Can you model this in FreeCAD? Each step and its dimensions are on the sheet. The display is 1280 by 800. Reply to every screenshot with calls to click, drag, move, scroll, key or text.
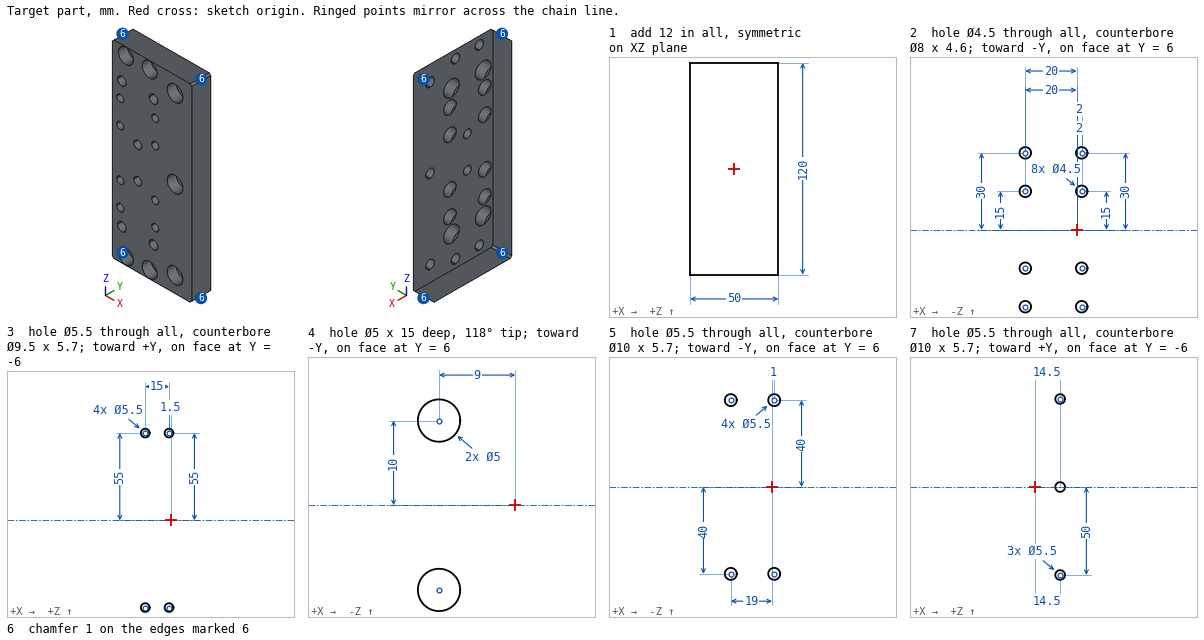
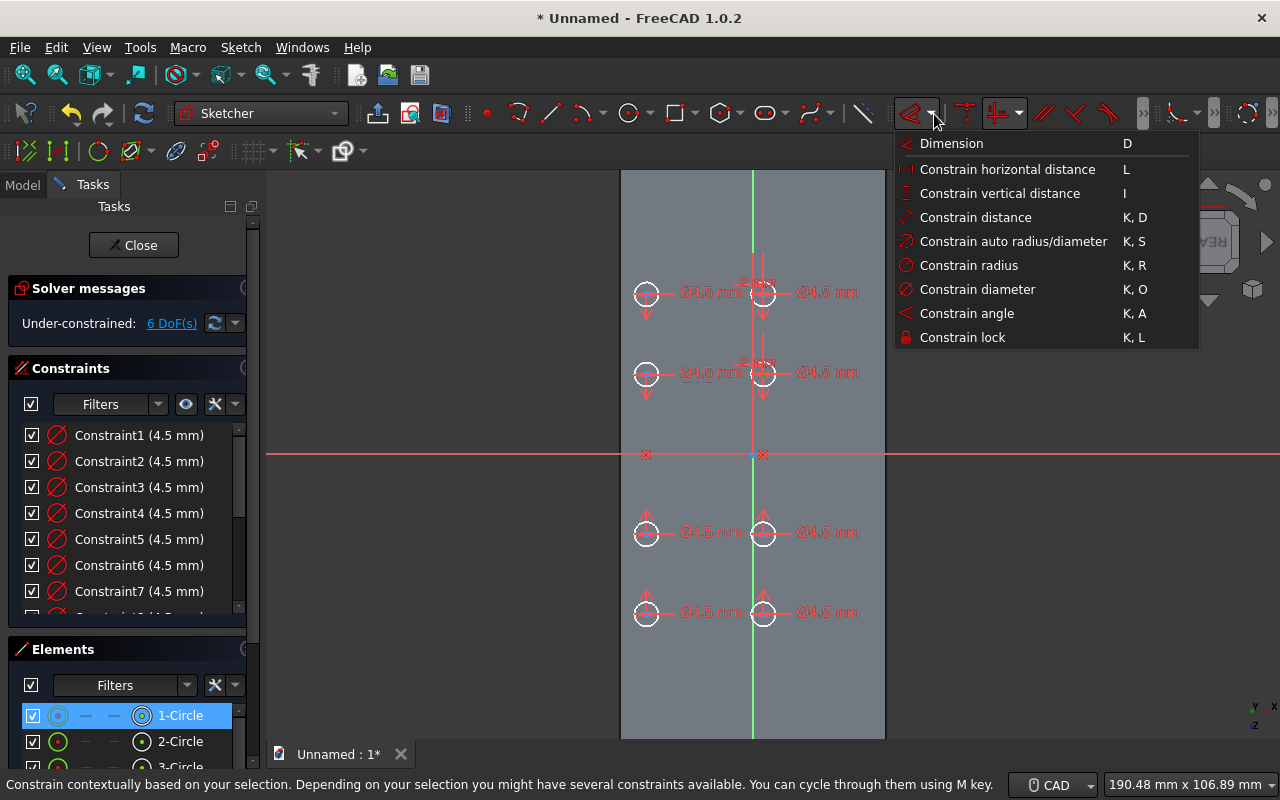
click(1047, 193)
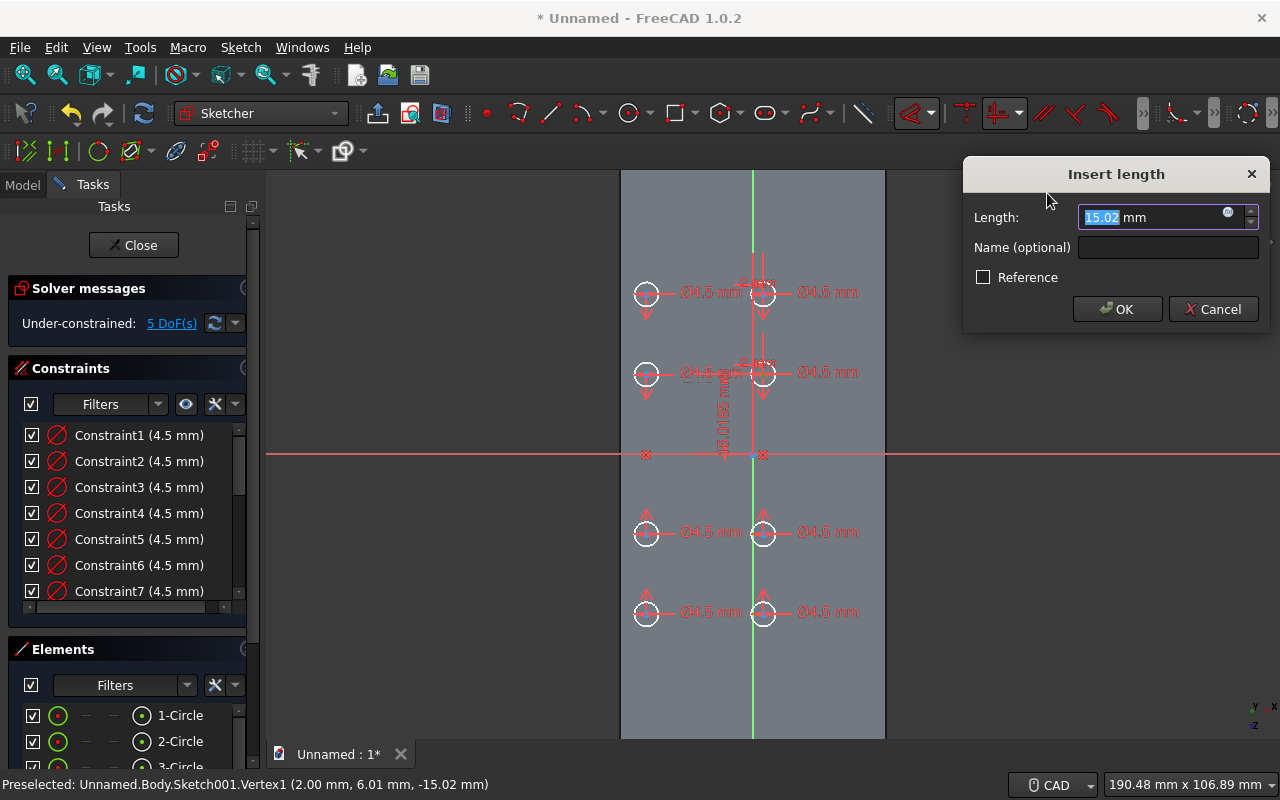
text(15)
key(Return)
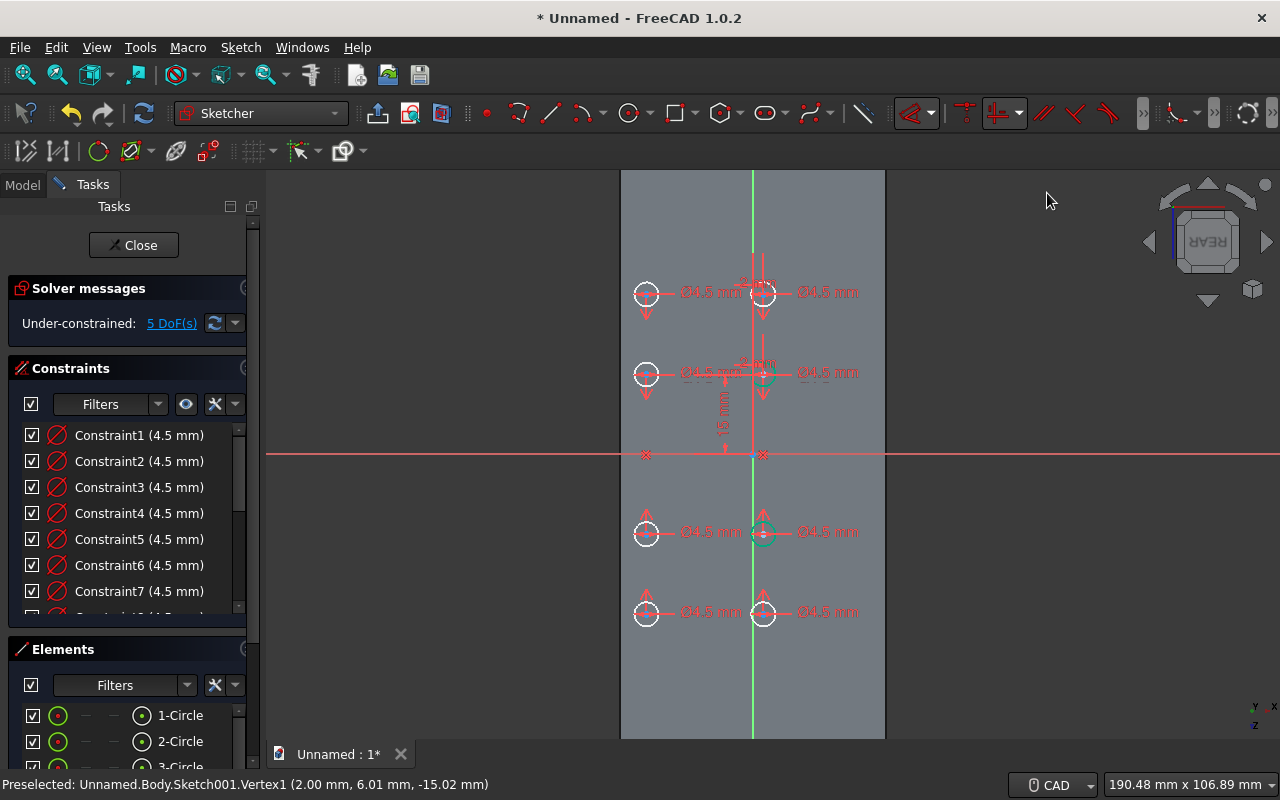
click(646, 294)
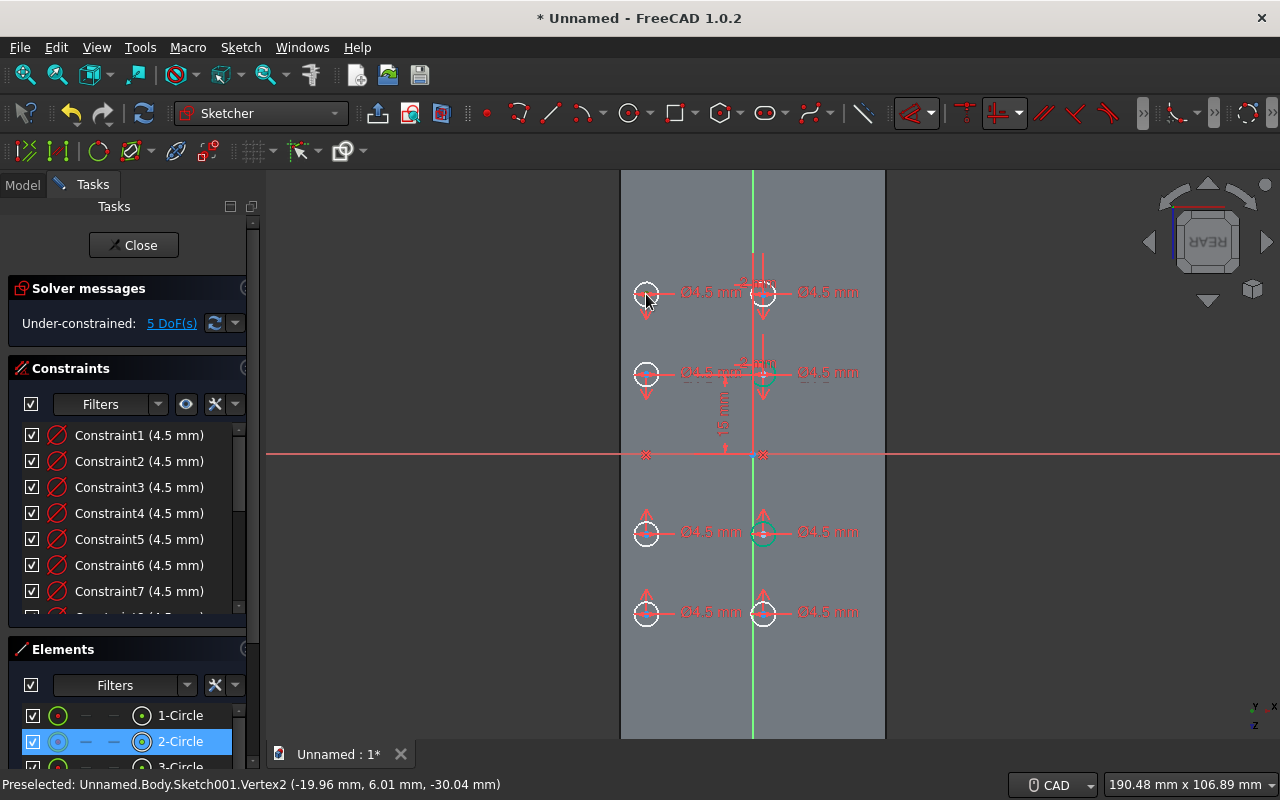
click(934, 114)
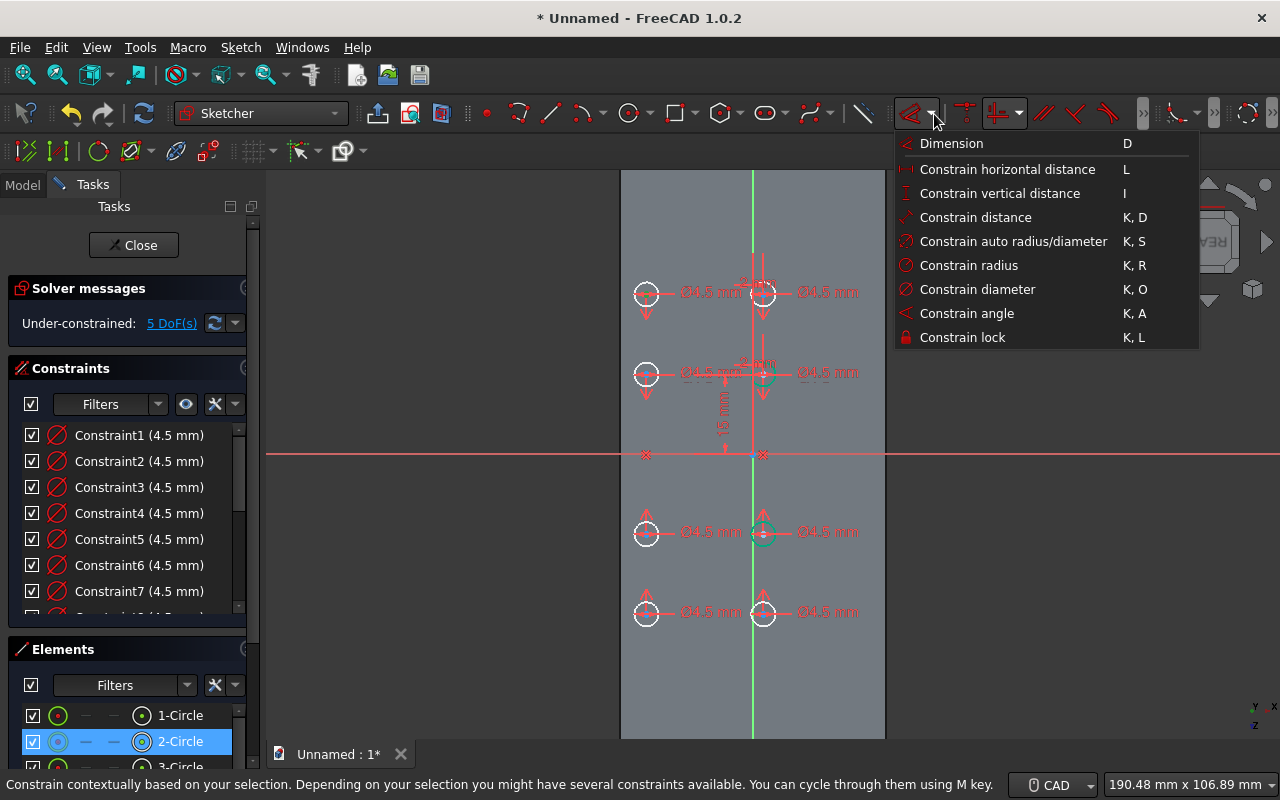
click(1047, 169)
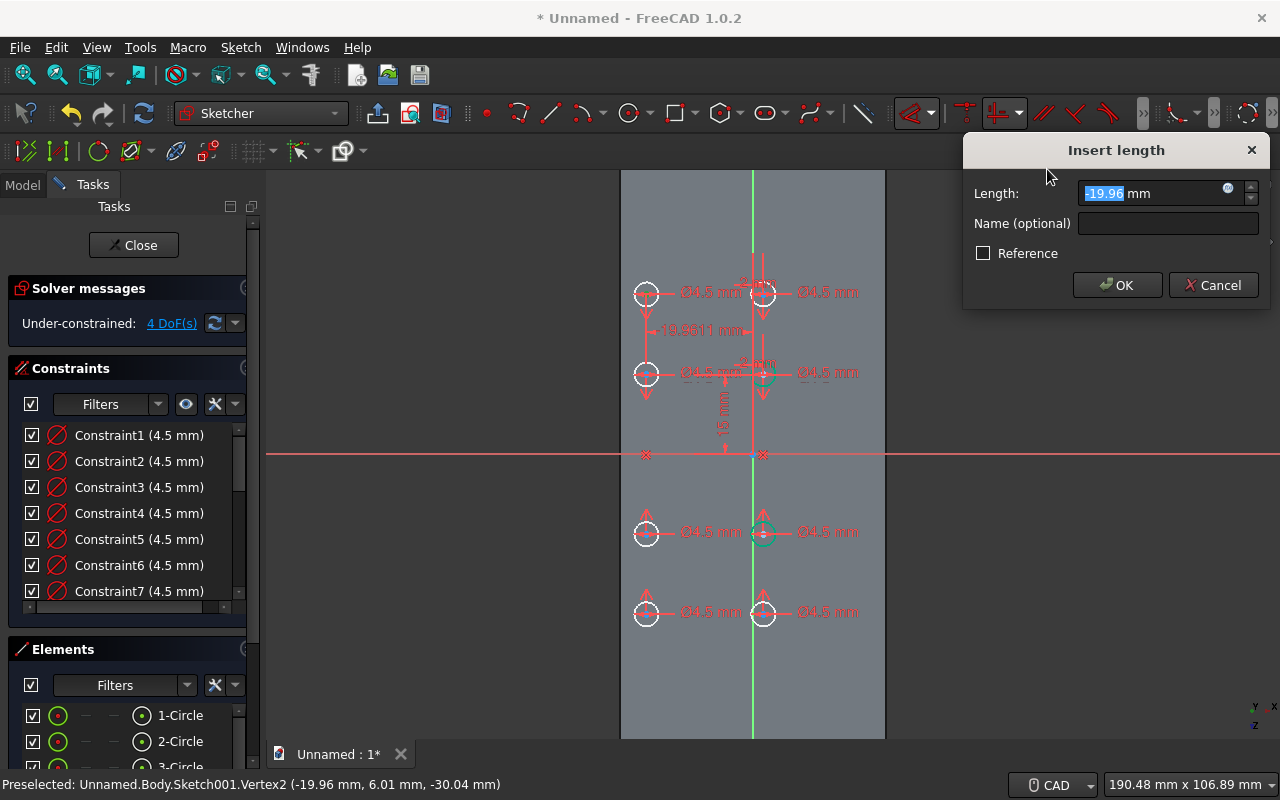
text(-20)
key(Return)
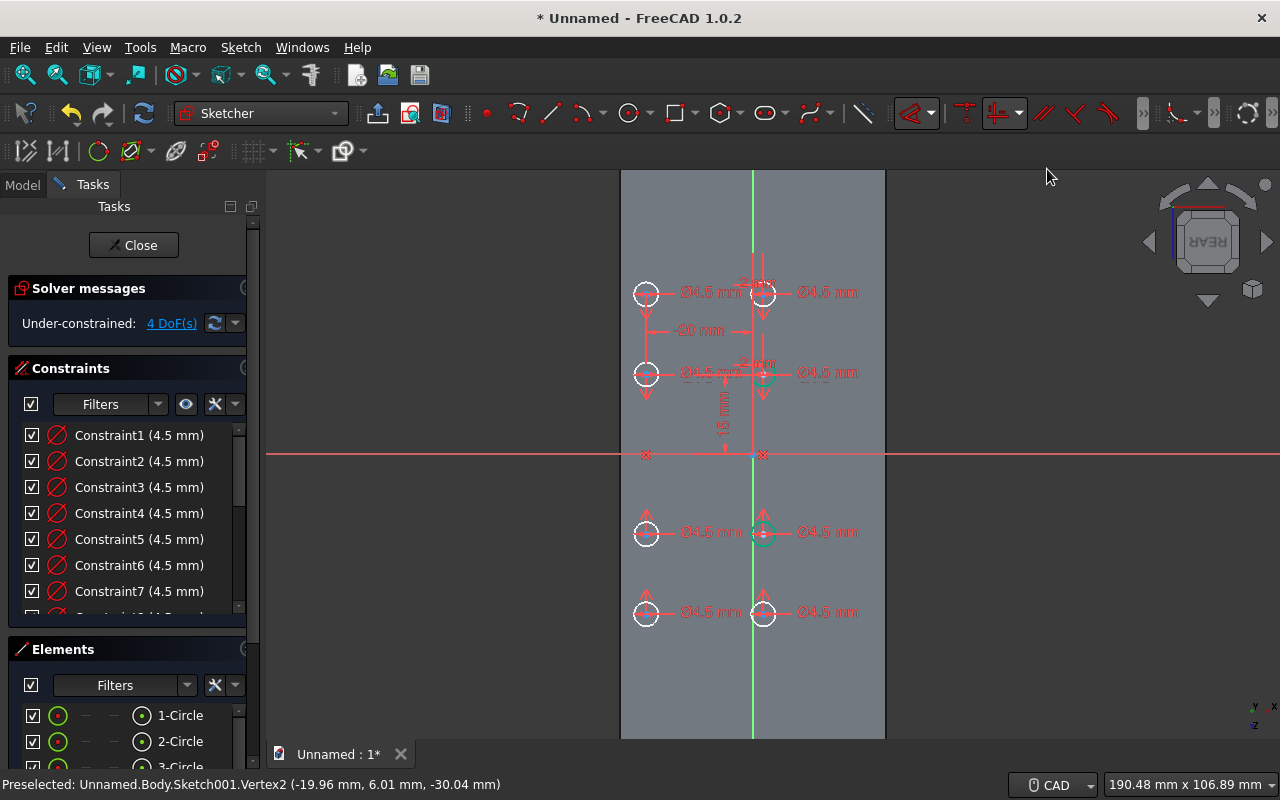
click(646, 294)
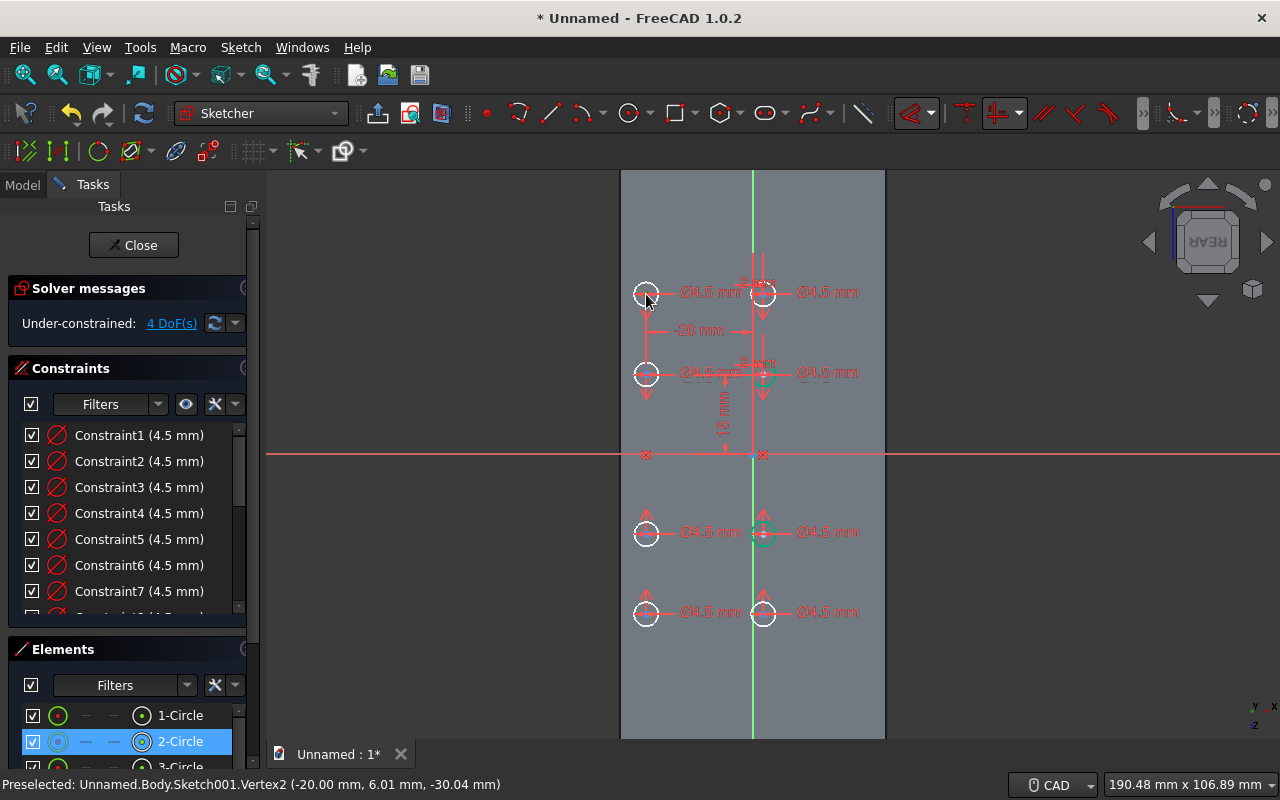
click(934, 114)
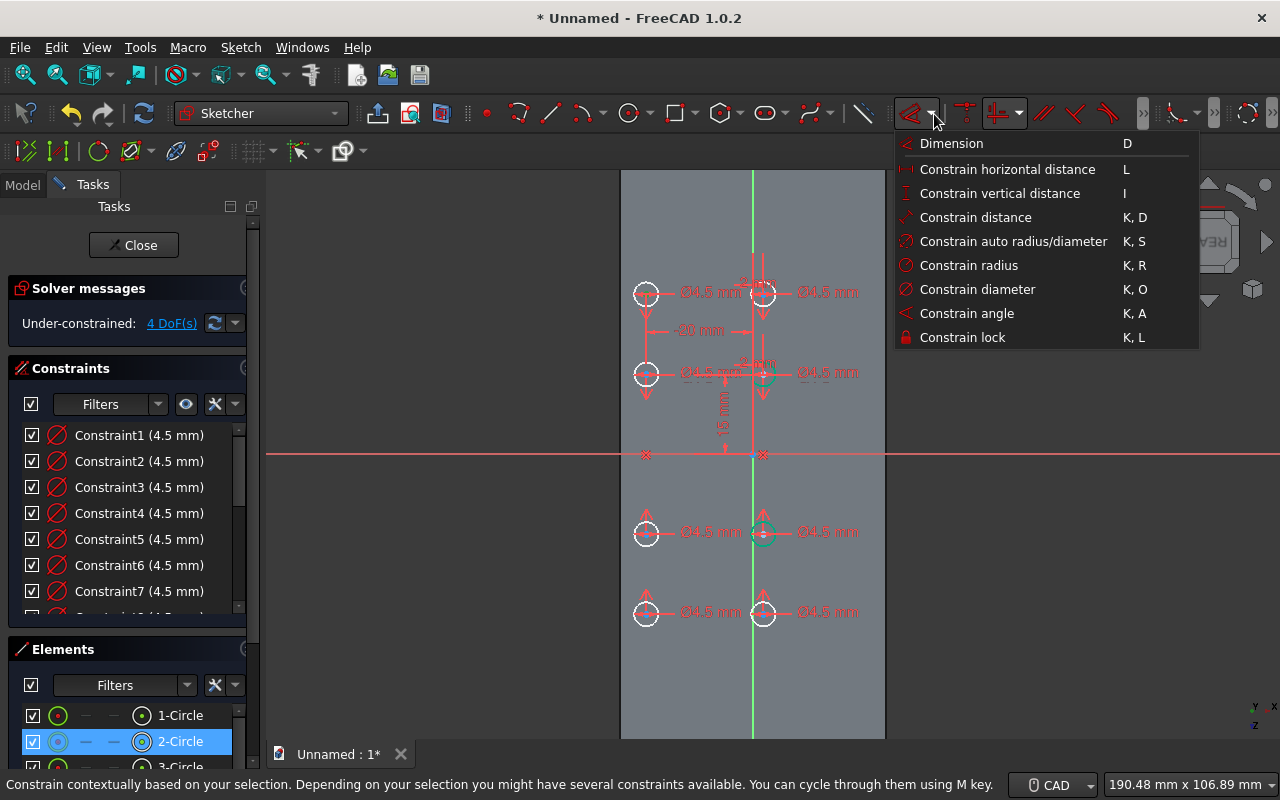
click(1047, 193)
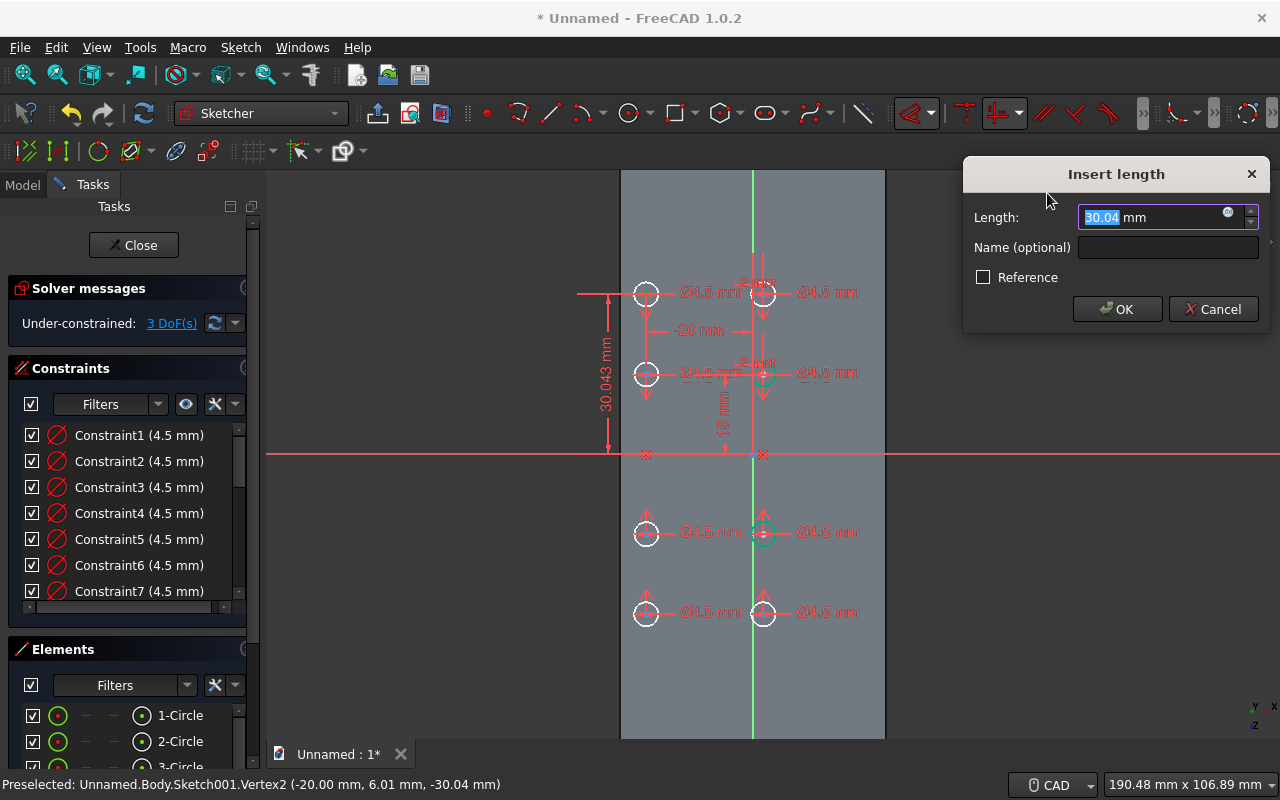
text(30)
key(Return)